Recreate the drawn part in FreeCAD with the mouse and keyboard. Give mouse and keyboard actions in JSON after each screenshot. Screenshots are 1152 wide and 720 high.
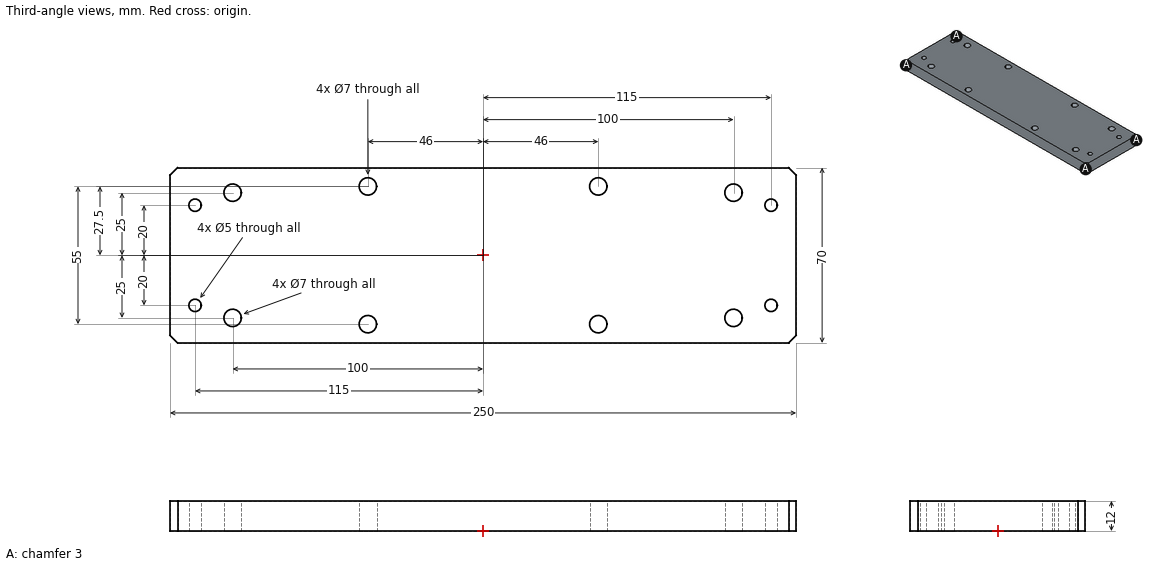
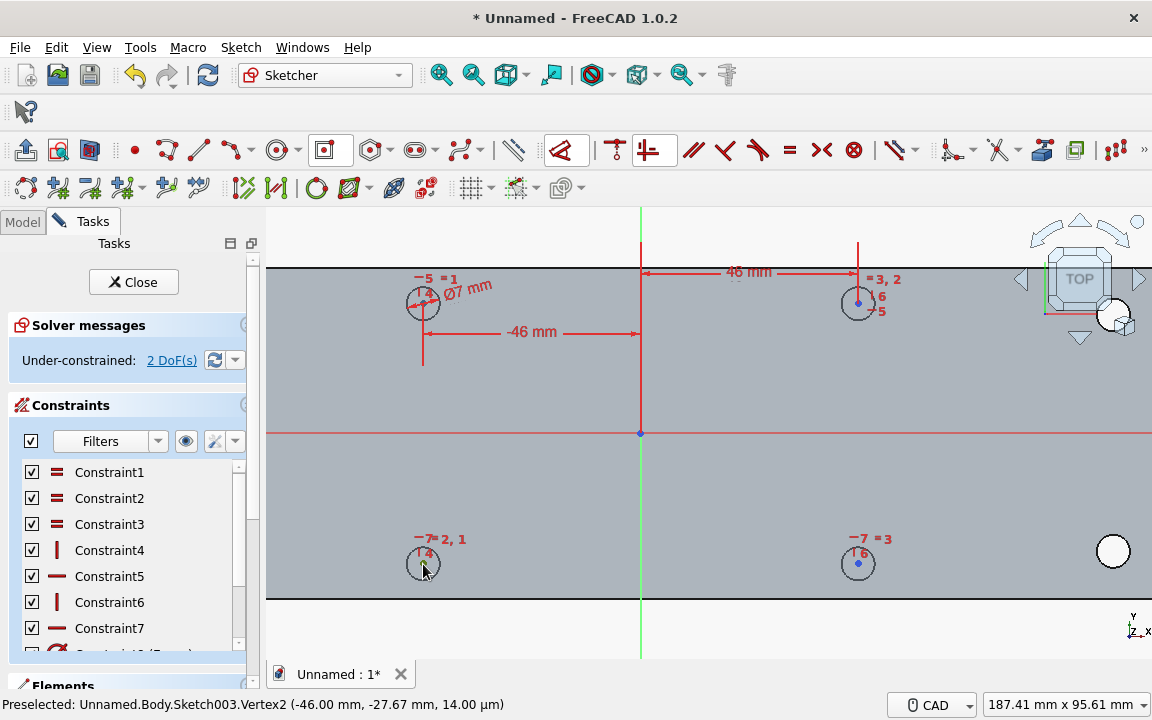
{"action": "left_click", "coordinate": [584, 150]}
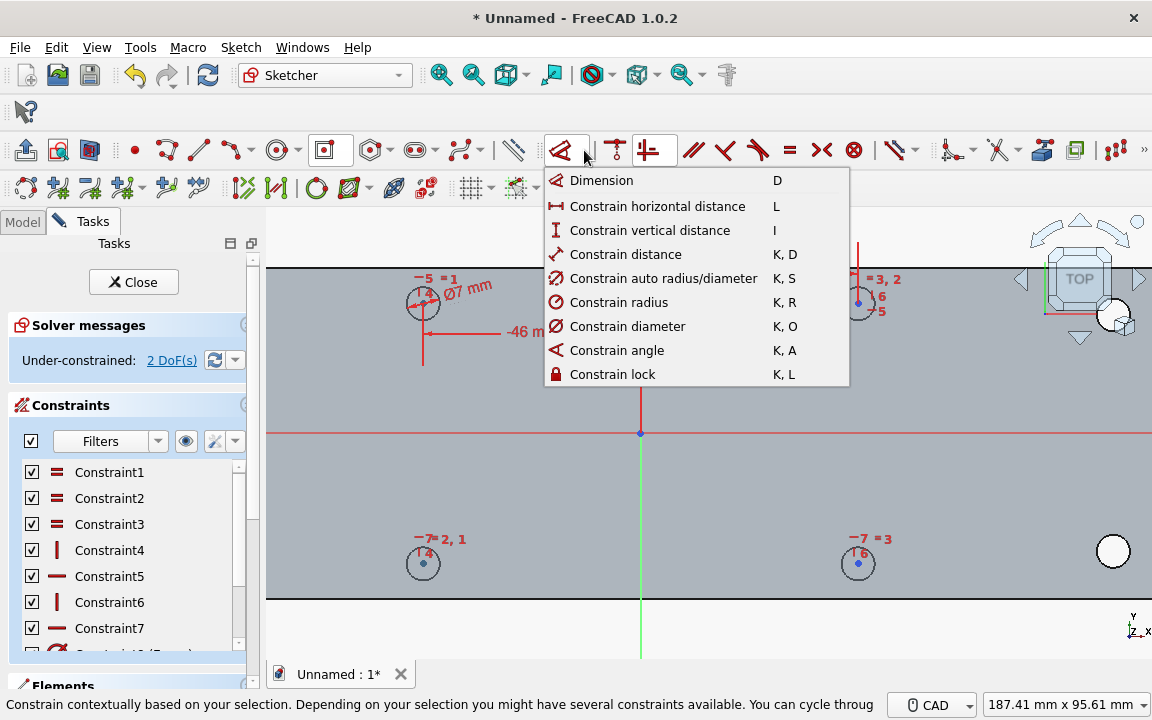
{"action": "left_click", "coordinate": [697, 230]}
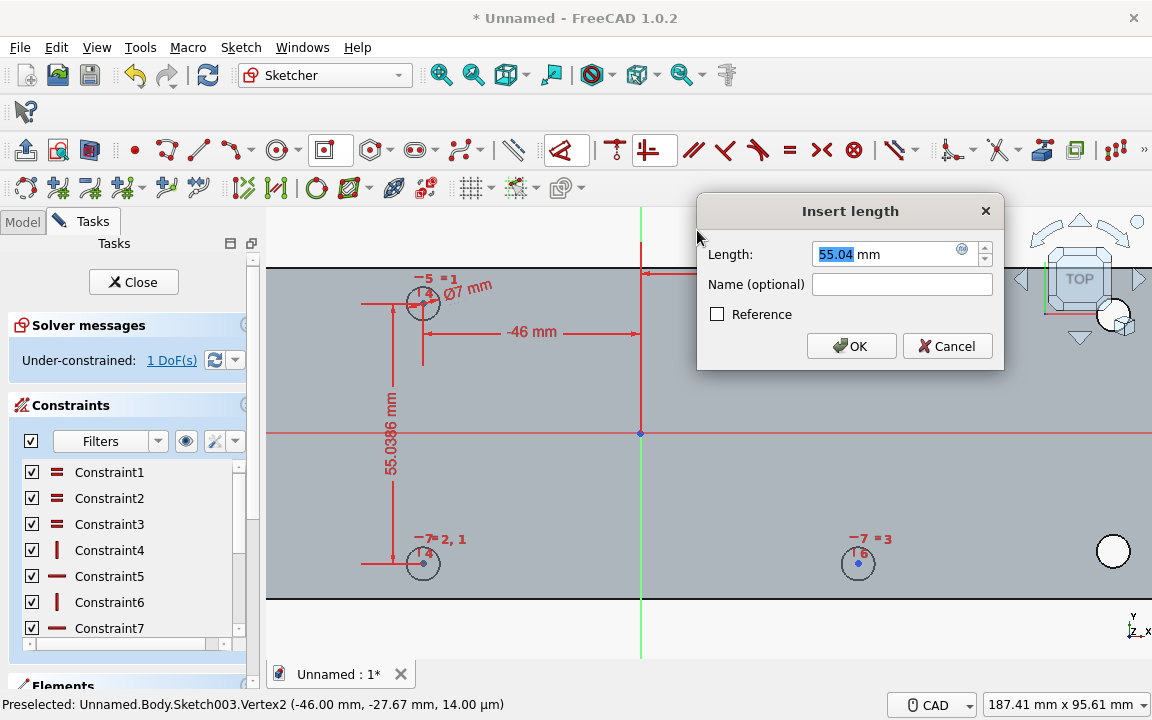
{"action": "type", "text": "55"}
{"action": "key", "text": "Return"}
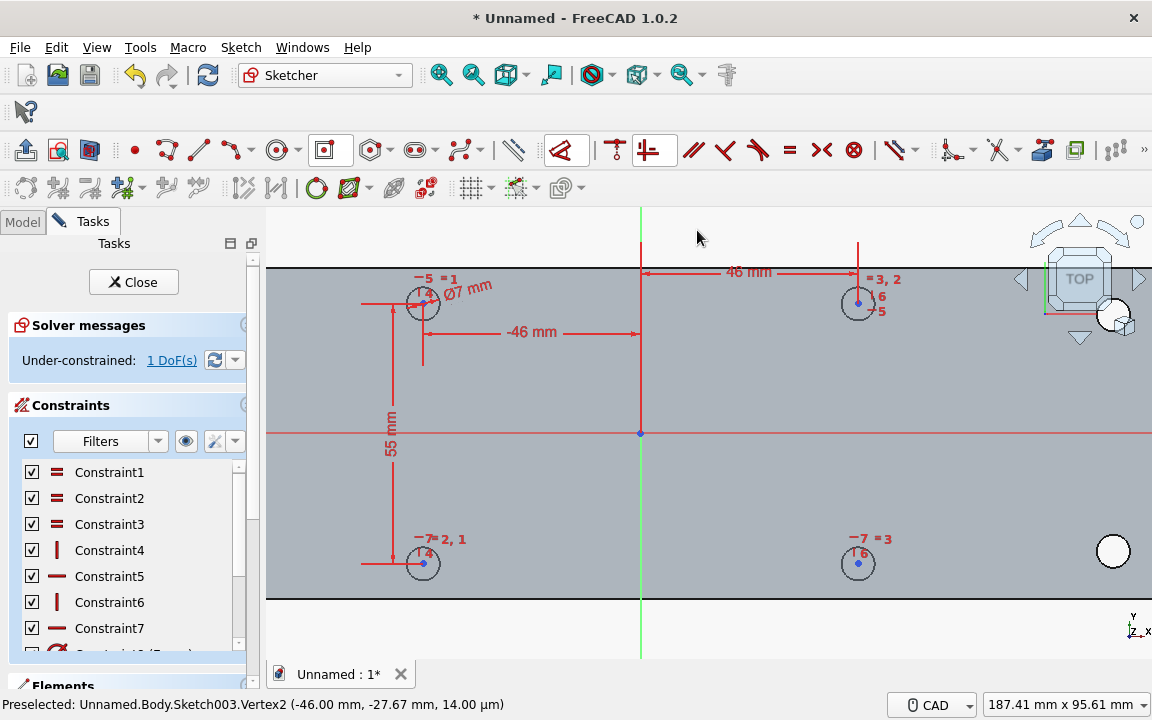
{"action": "left_click", "coordinate": [423, 304]}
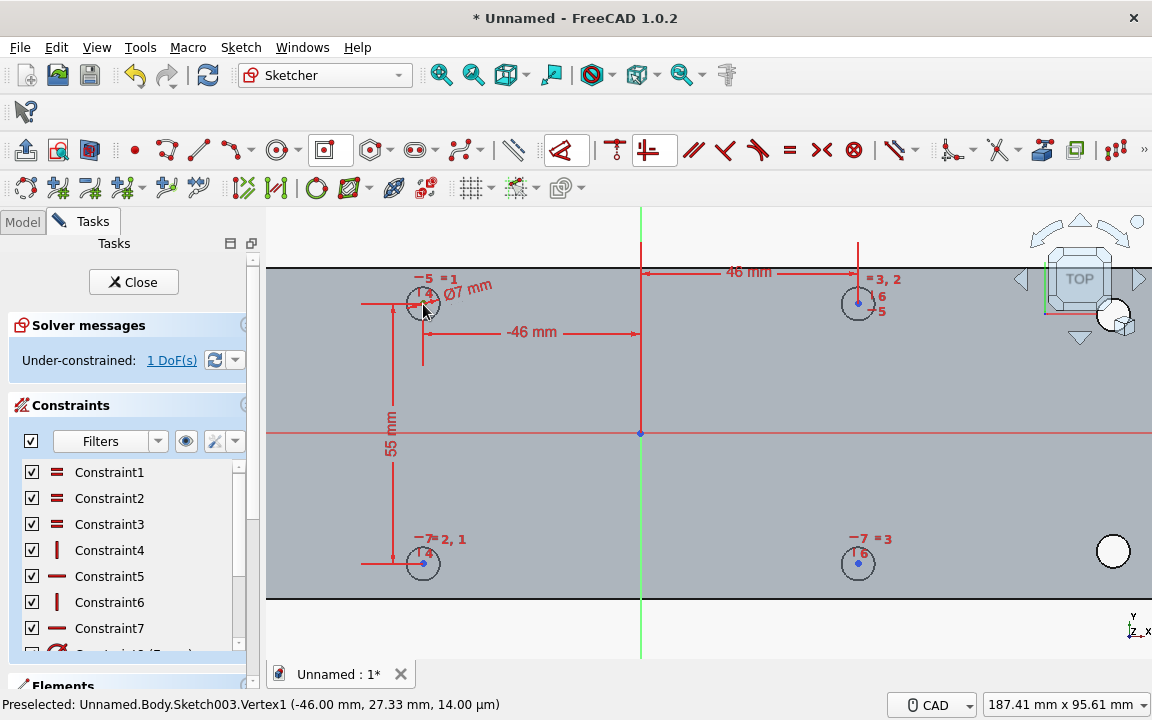
{"action": "key", "text": "i"}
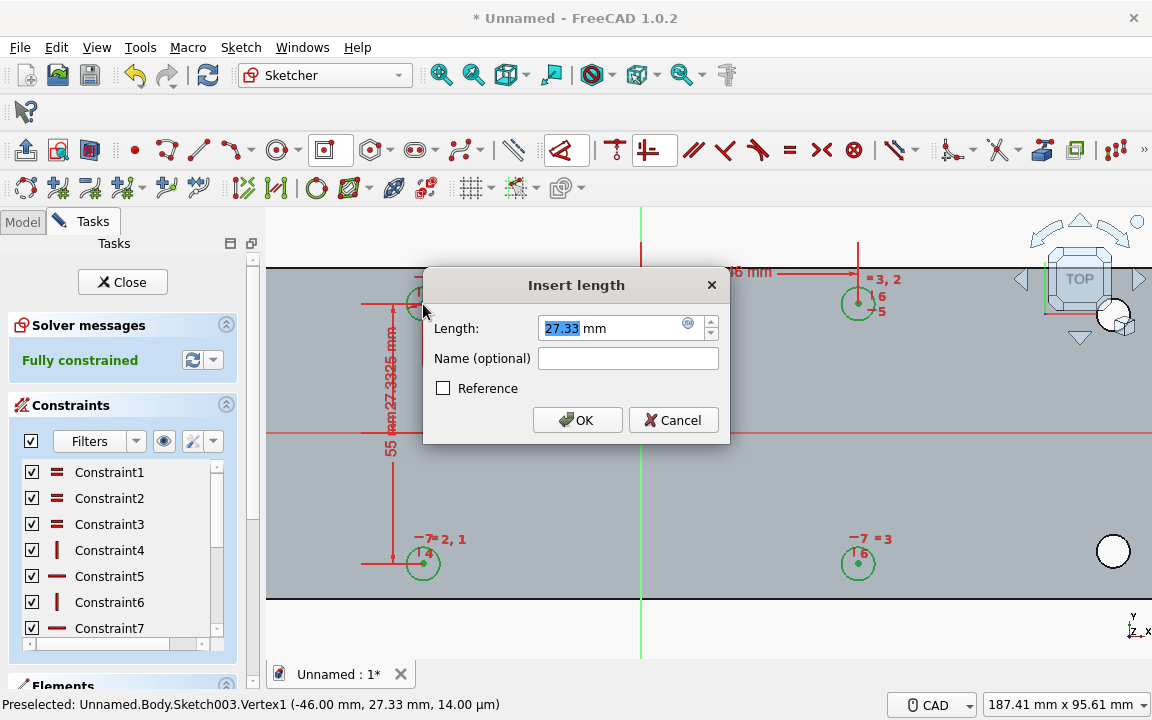
{"action": "type", "text": "27.5"}
{"action": "key", "text": "Return"}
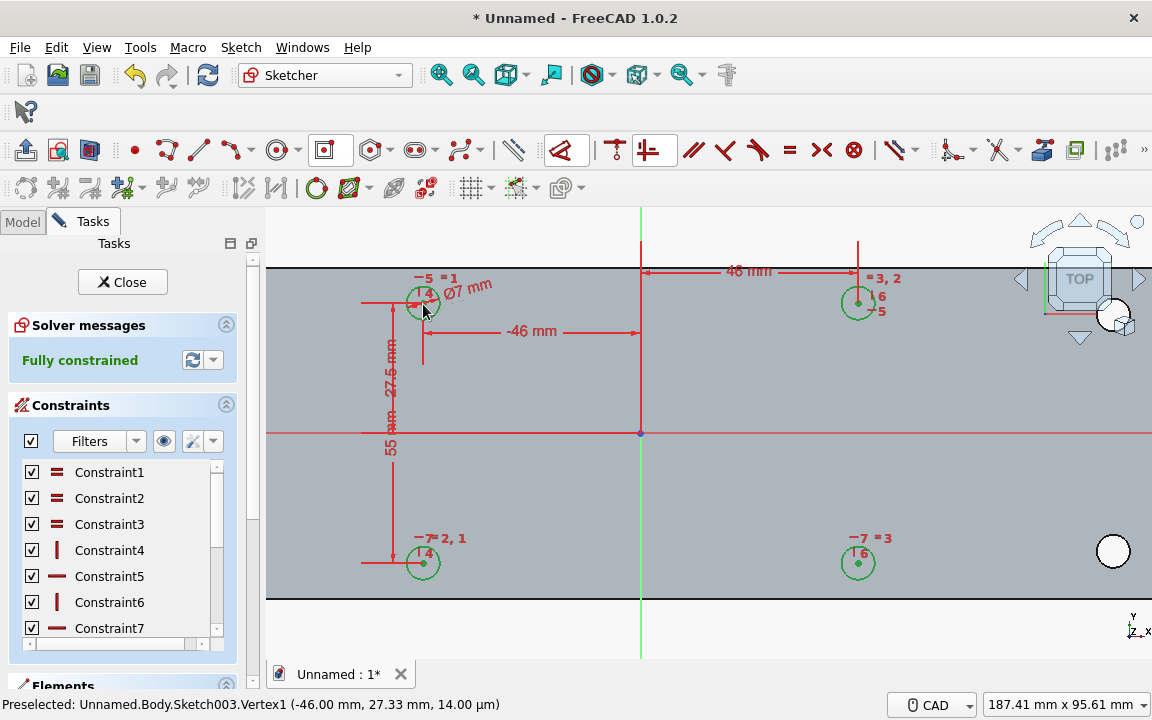
{"action": "left_click", "coordinate": [123, 282]}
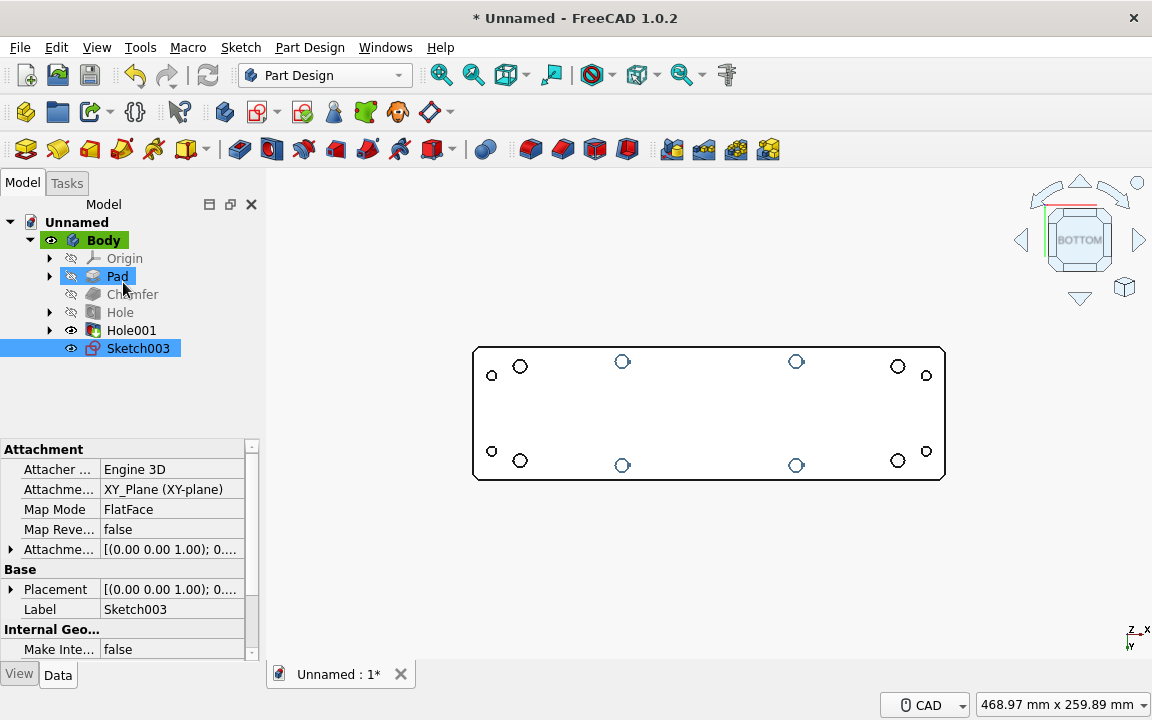
{"action": "left_click", "coordinate": [272, 150]}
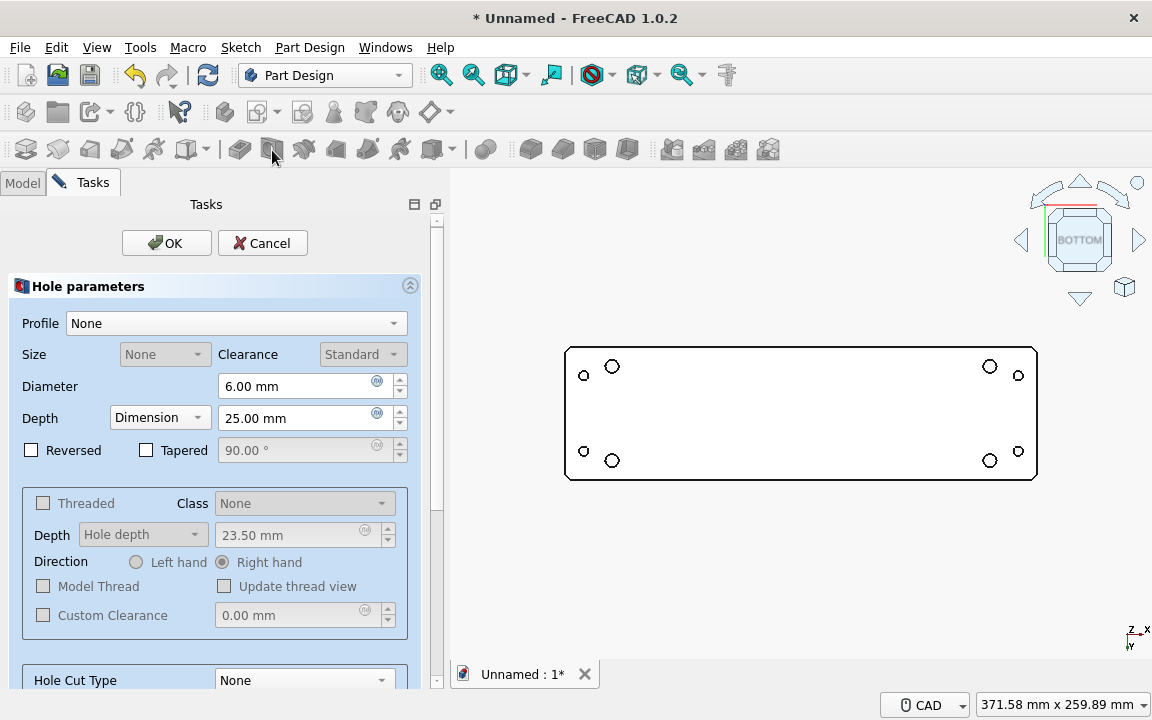
{"action": "triple_click", "coordinate": [305, 386]}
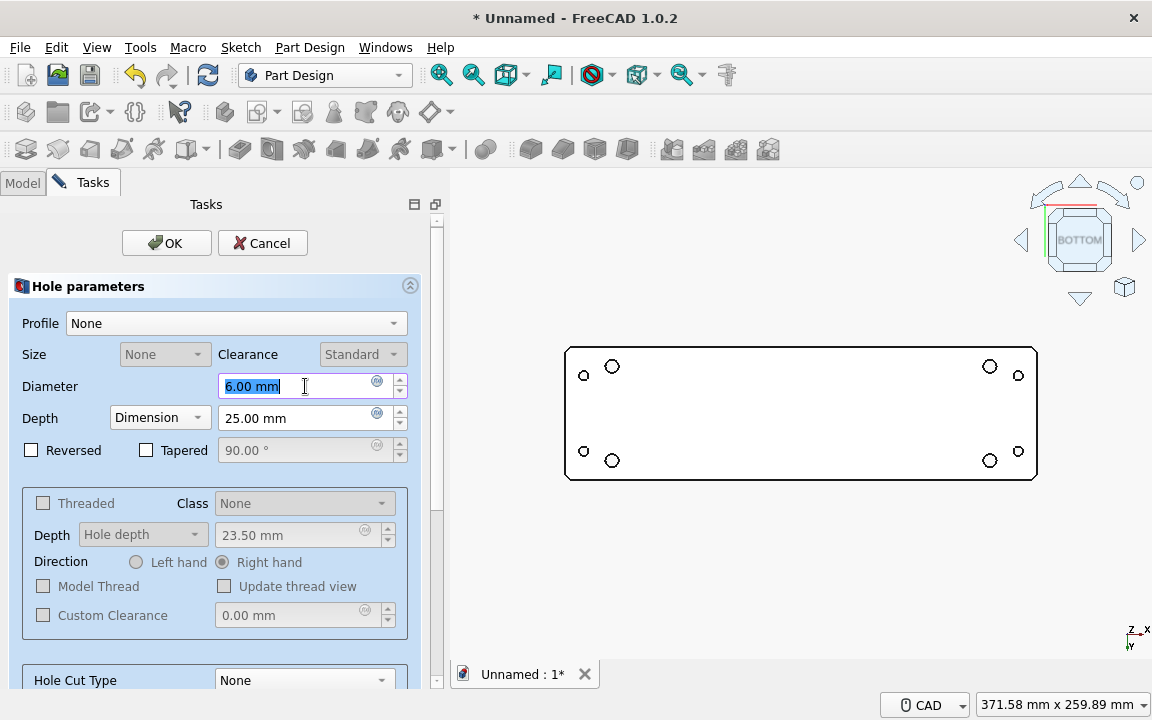
{"action": "type", "text": "7"}
{"action": "key", "text": "Tab"}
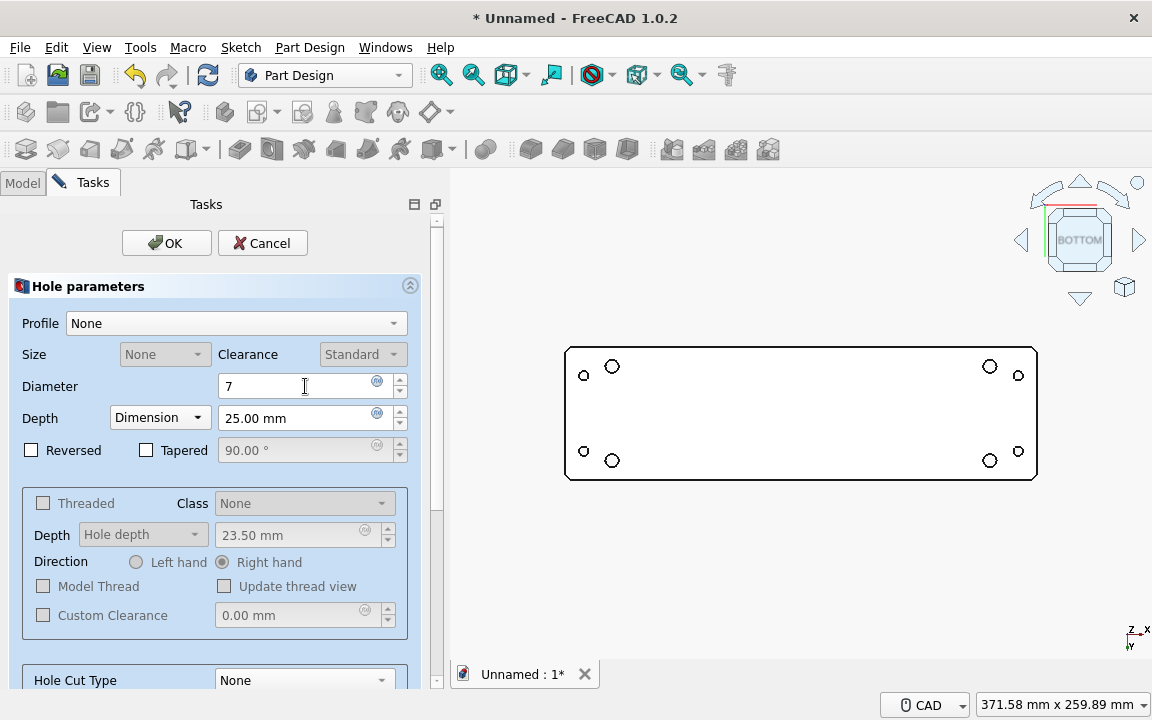
{"action": "left_click", "coordinate": [161, 418]}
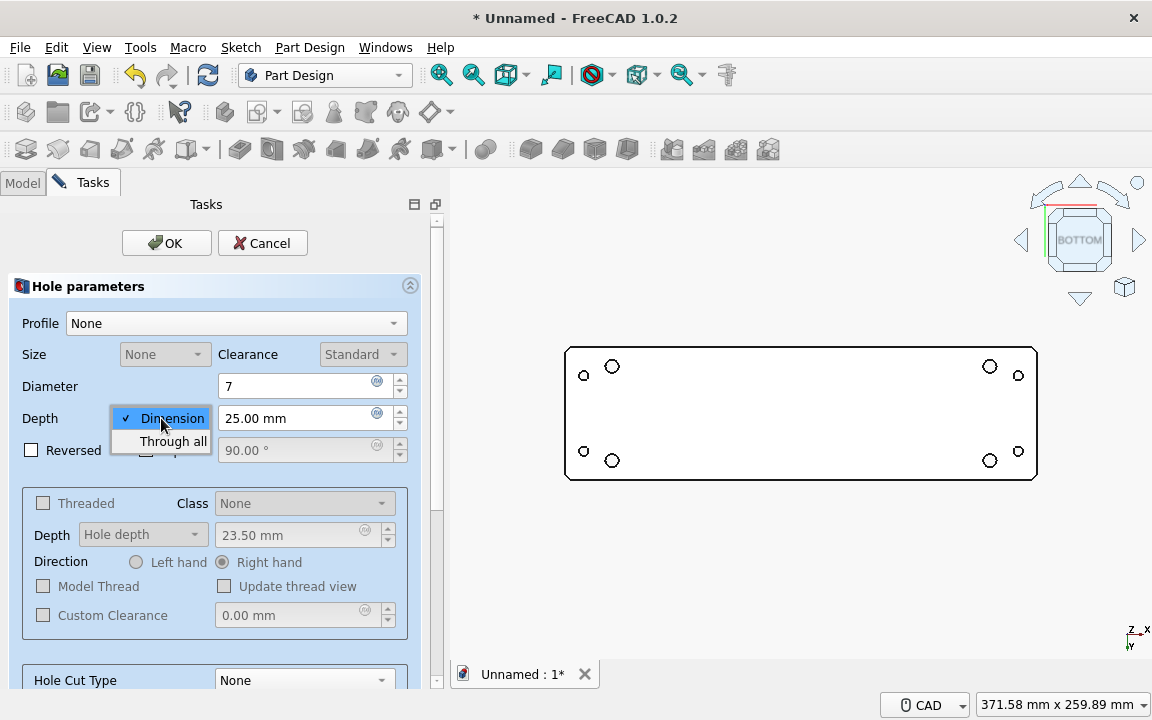
{"action": "left_click", "coordinate": [160, 442]}